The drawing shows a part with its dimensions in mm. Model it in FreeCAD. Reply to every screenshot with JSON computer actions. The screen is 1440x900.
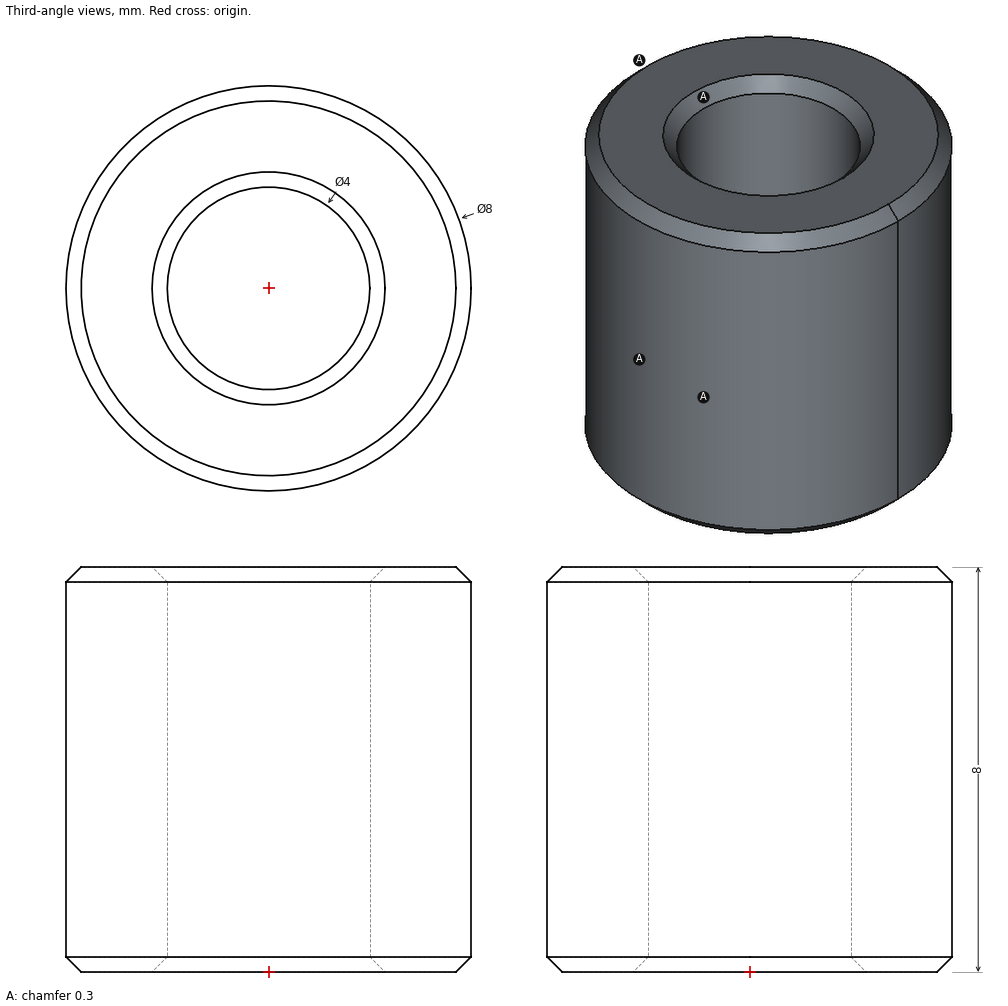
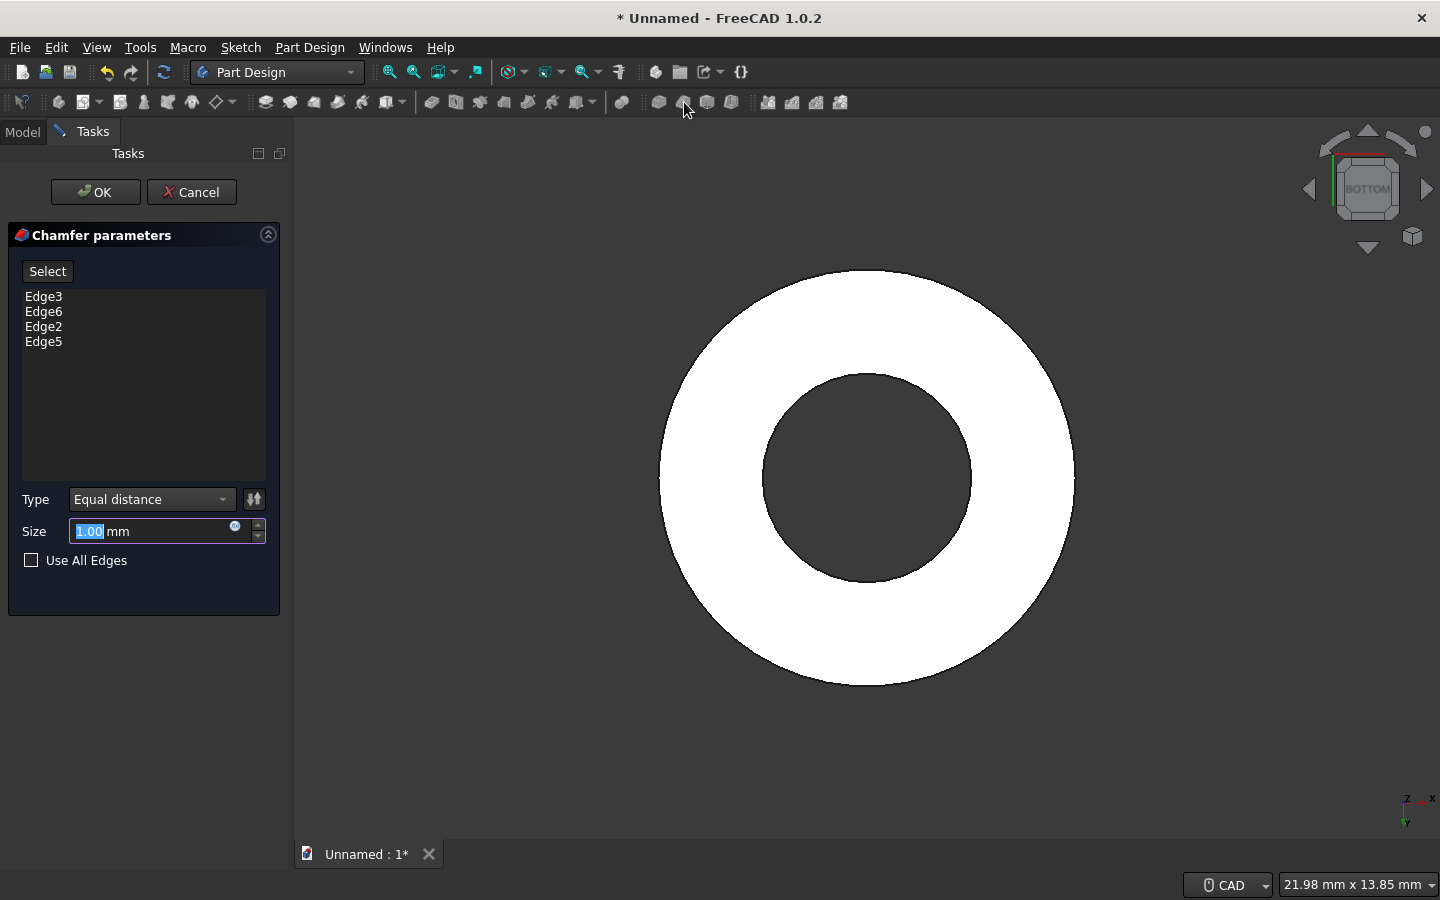
{"action": "type", "text": "0.3"}
{"action": "key", "text": "Tab"}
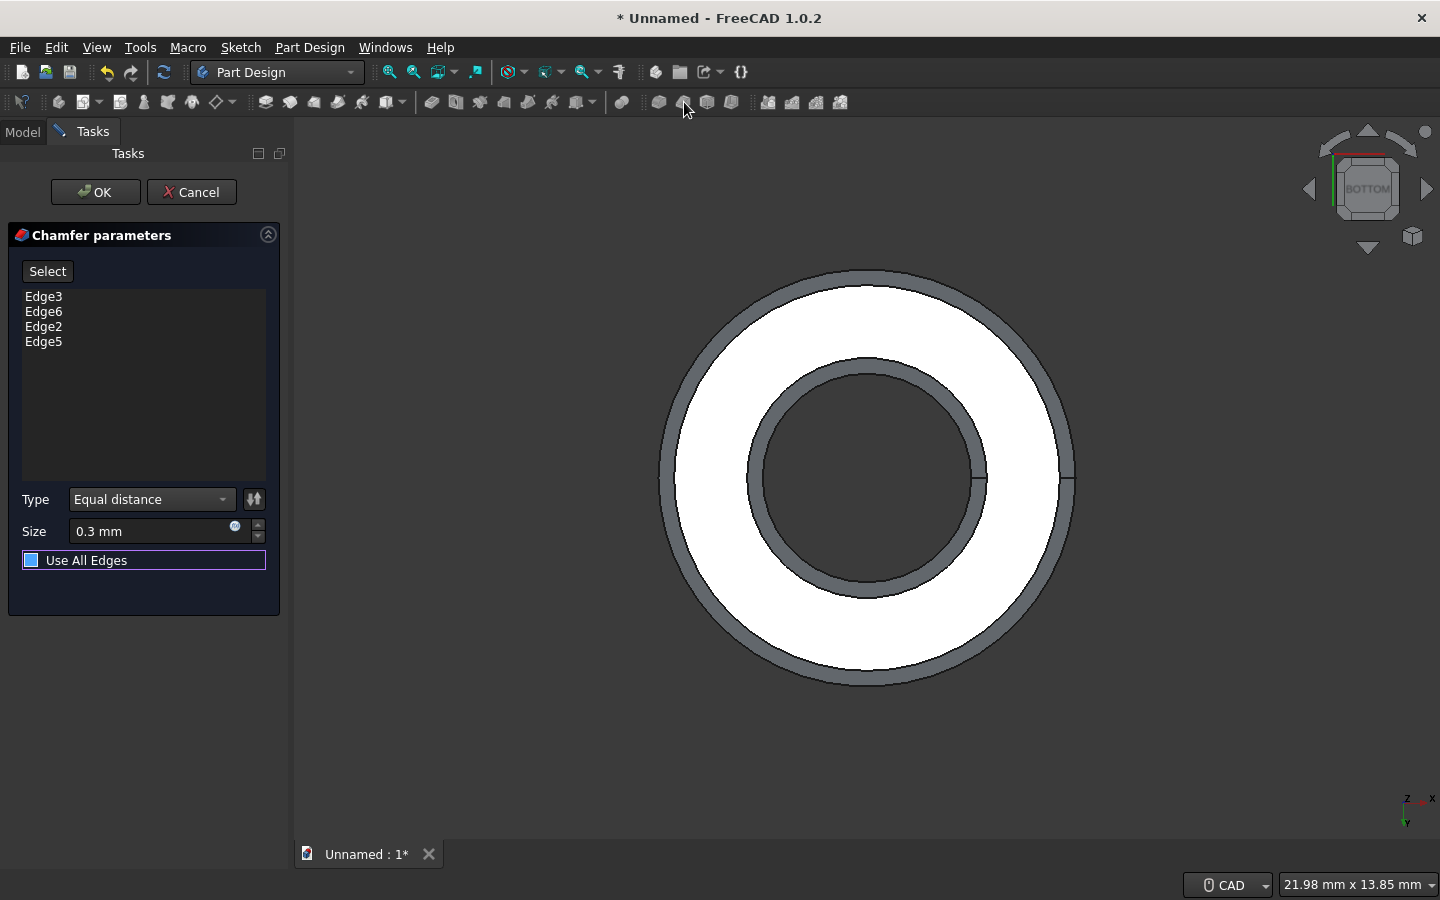
{"action": "left_click", "coordinate": [96, 192]}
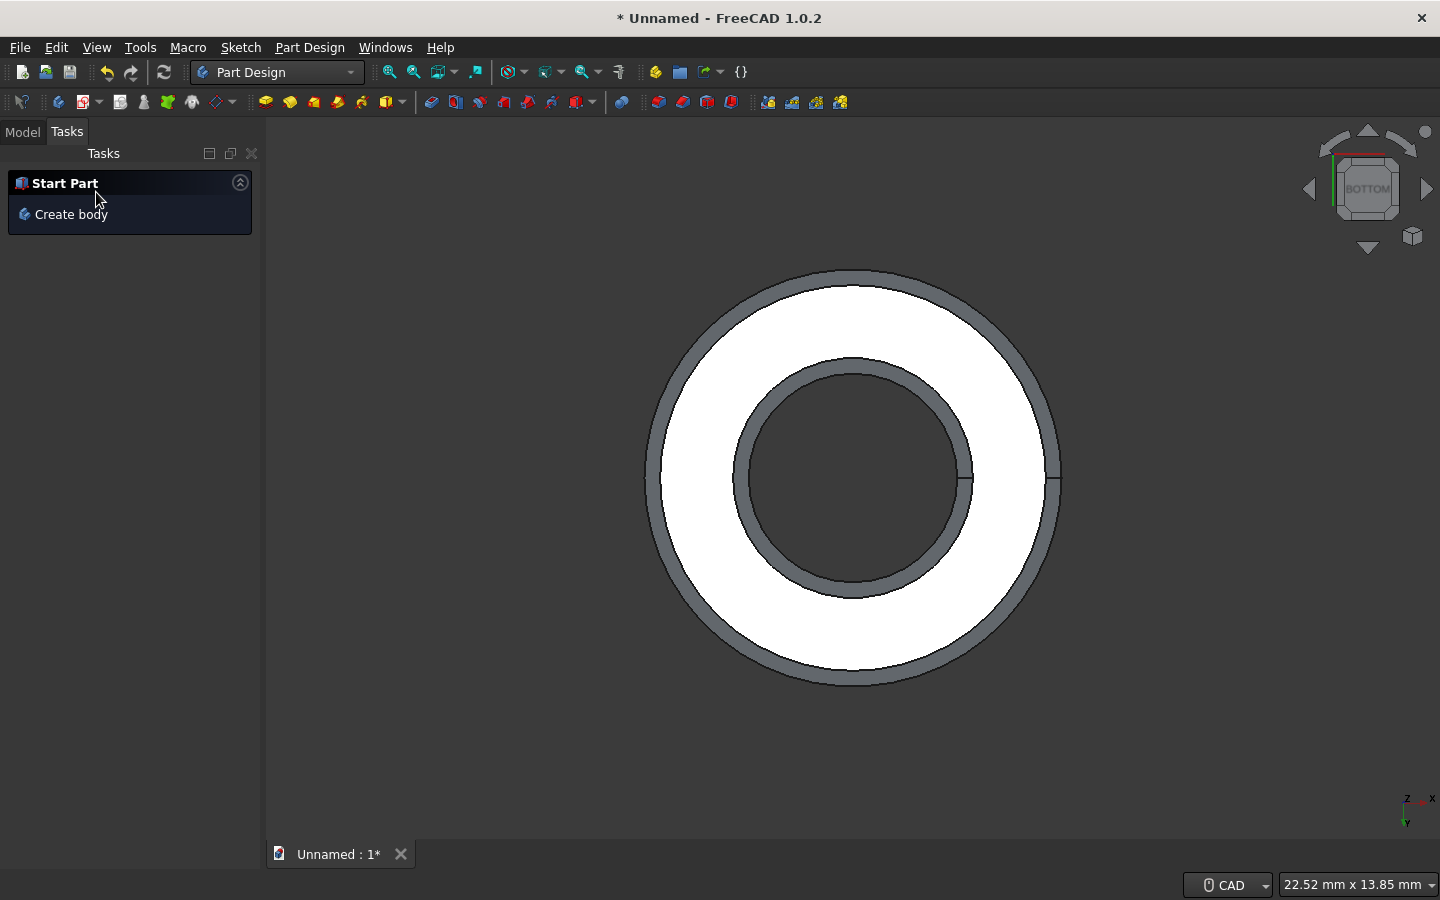
{"action": "key", "text": "0"}